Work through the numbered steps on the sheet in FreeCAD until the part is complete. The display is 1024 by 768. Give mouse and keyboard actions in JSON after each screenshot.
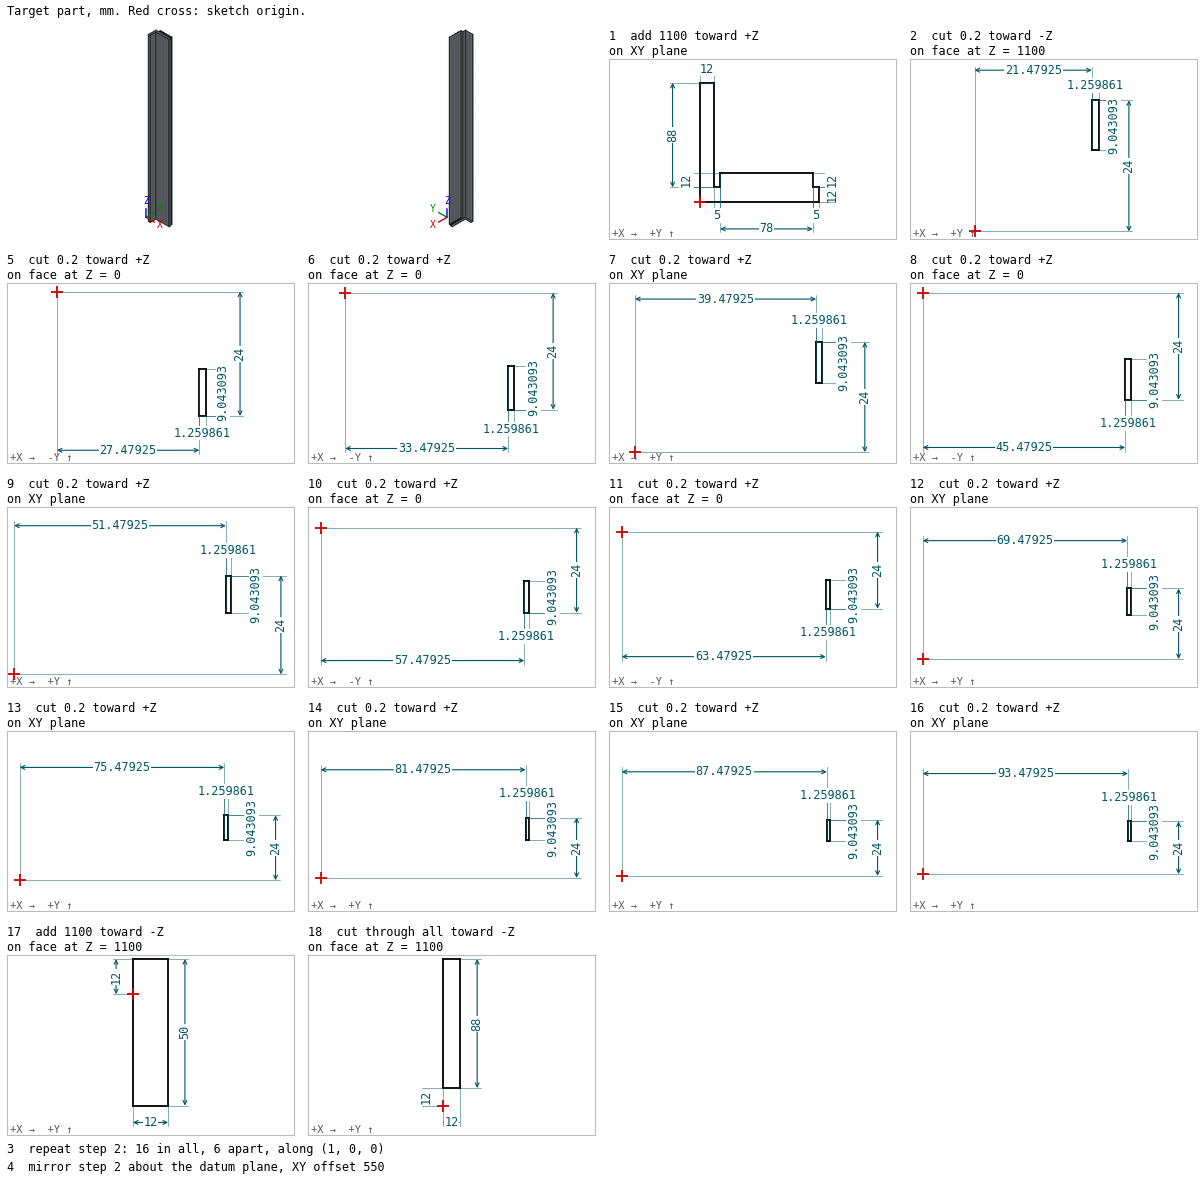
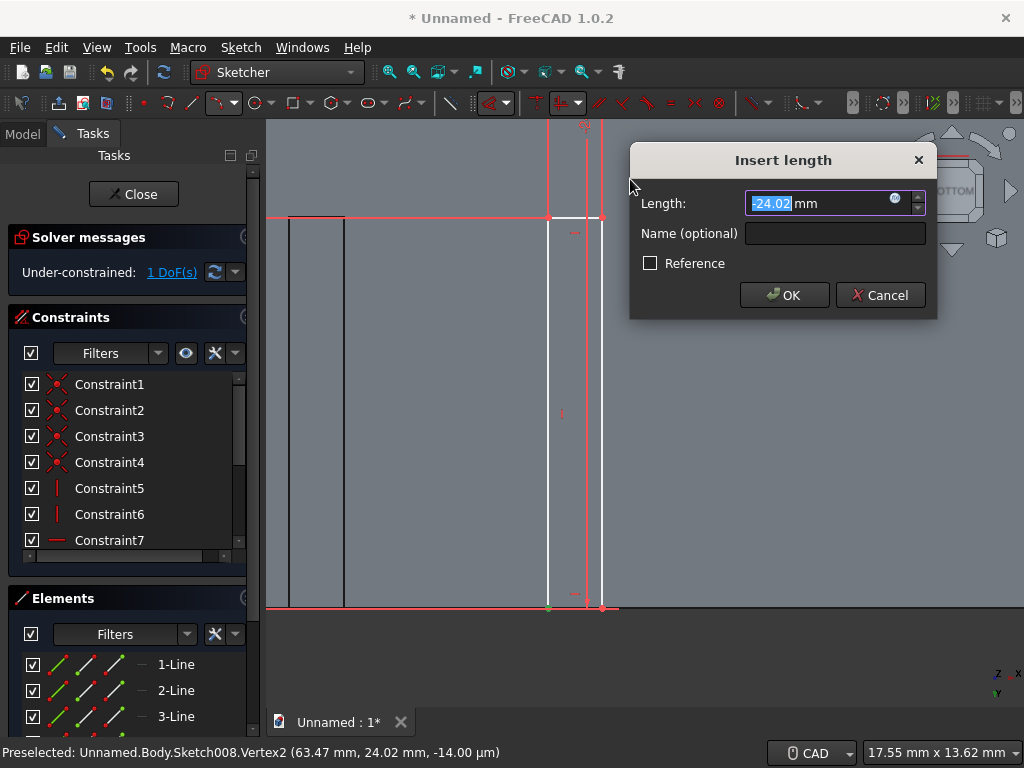
{"action": "type", "text": "-24"}
{"action": "key", "text": "Return"}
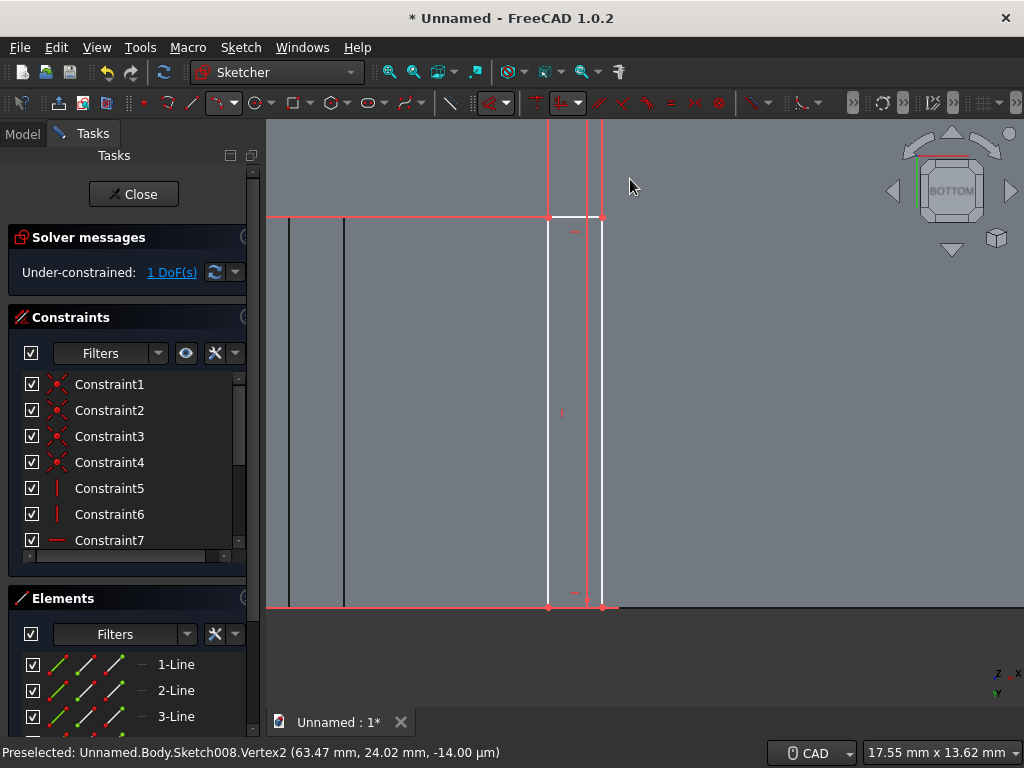
{"action": "left_click", "coordinate": [548, 217]}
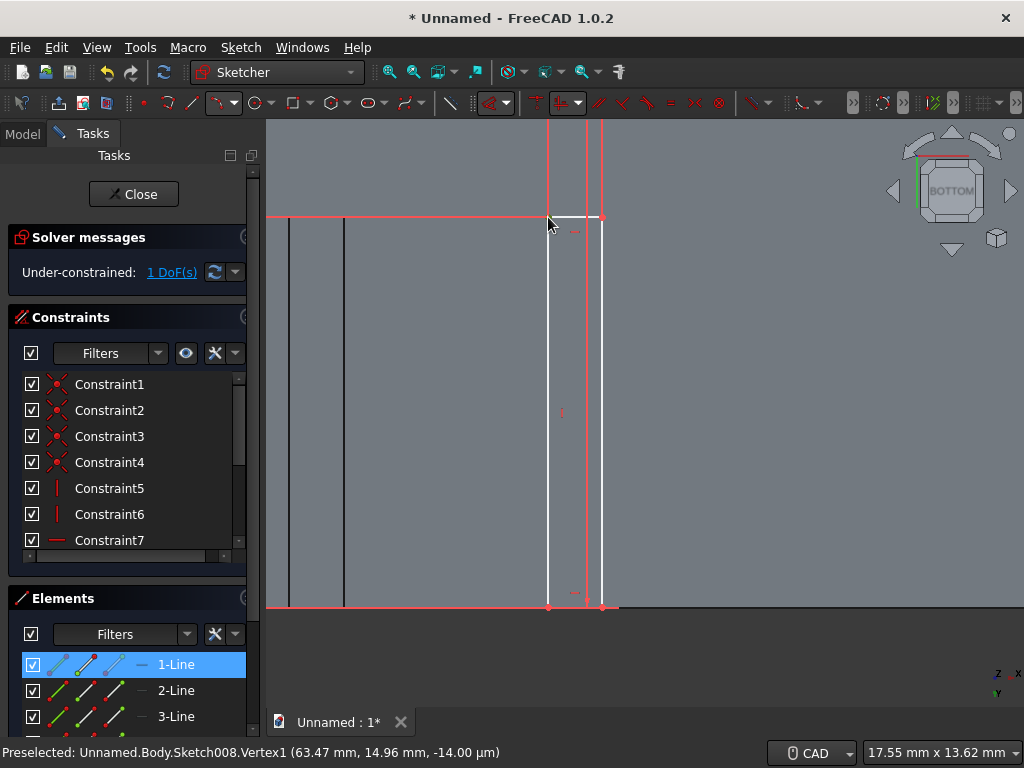
{"action": "key", "text": "l"}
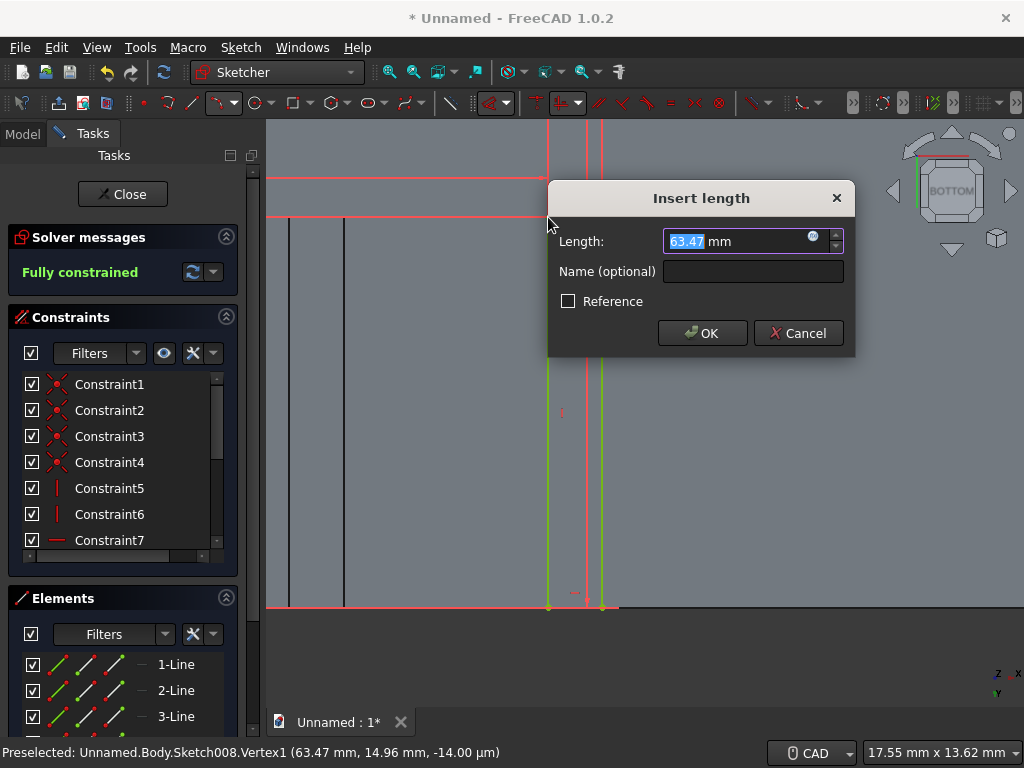
{"action": "type", "text": "63.47925"}
{"action": "key", "text": "Return"}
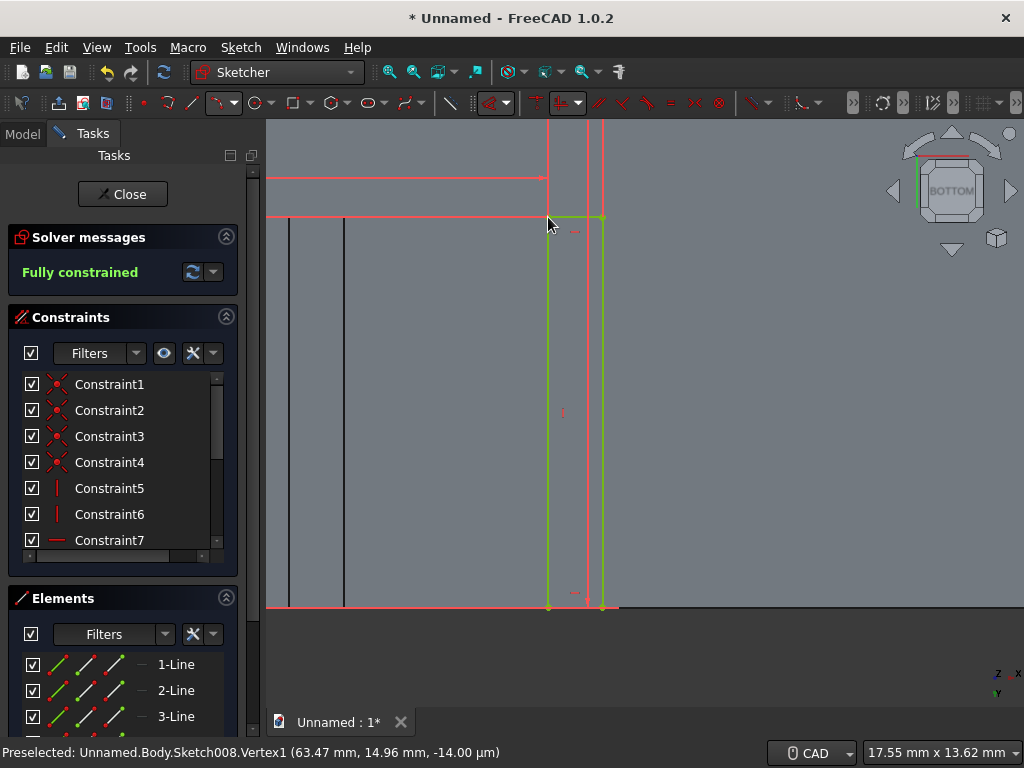
{"action": "left_click", "coordinate": [123, 194]}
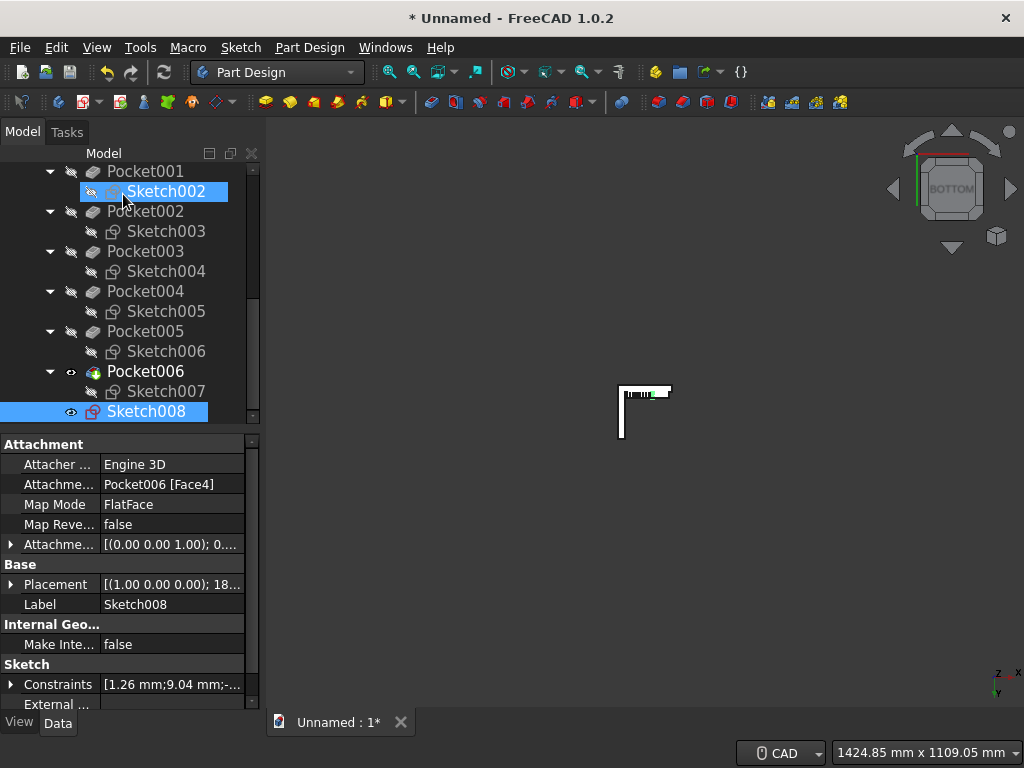
{"action": "left_click", "coordinate": [432, 102]}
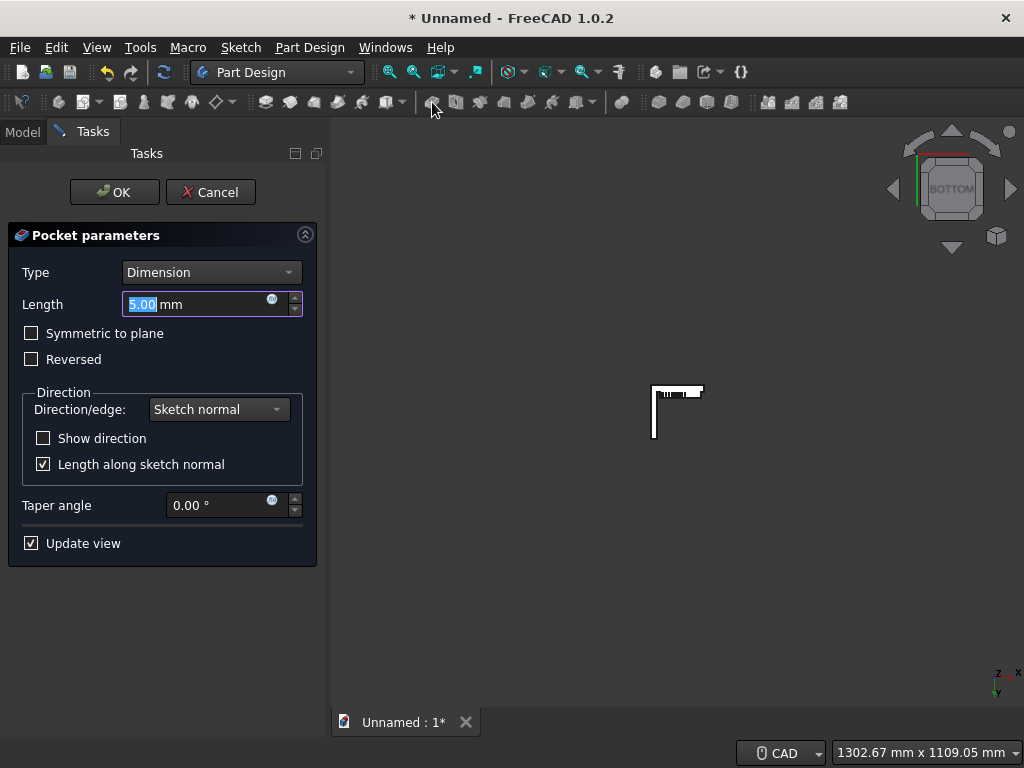
{"action": "type", "text": "0.2"}
{"action": "key", "text": "Tab"}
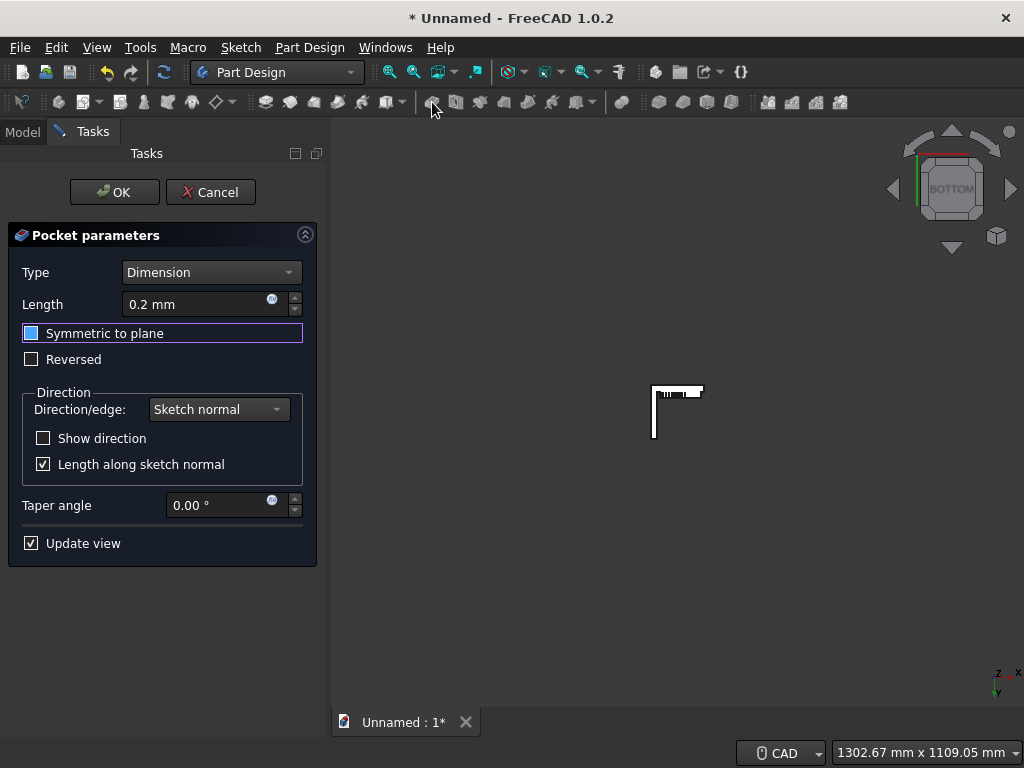
{"action": "left_click", "coordinate": [115, 192]}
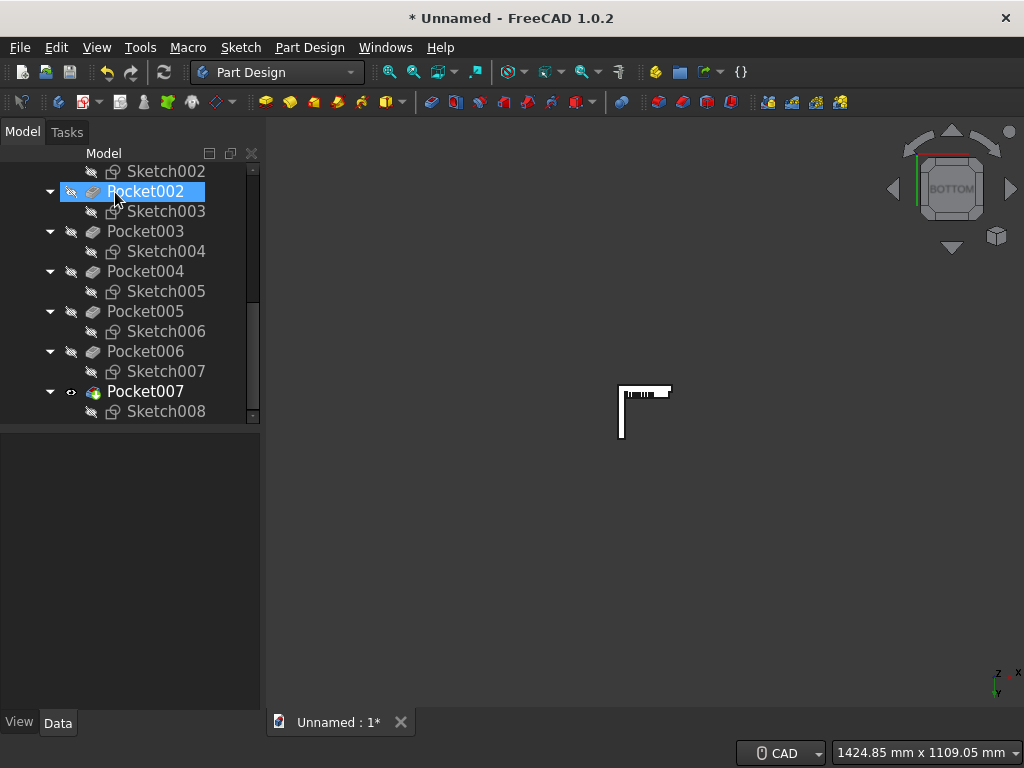
{"action": "key", "text": "v f"}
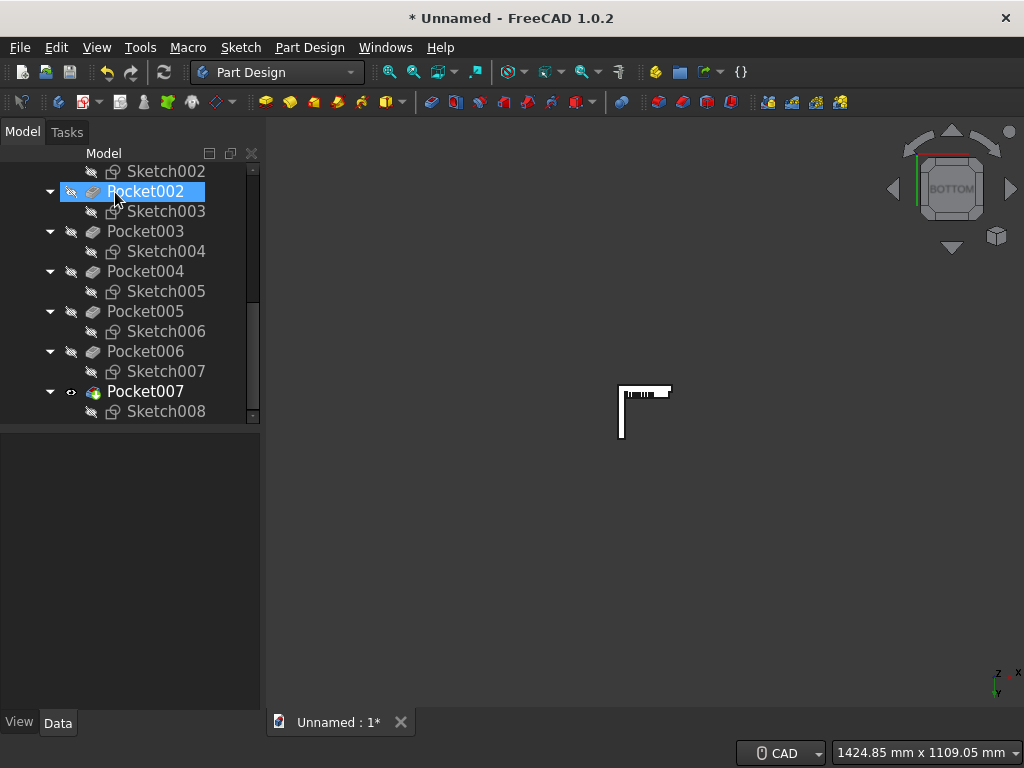
{"action": "left_click", "coordinate": [84, 102]}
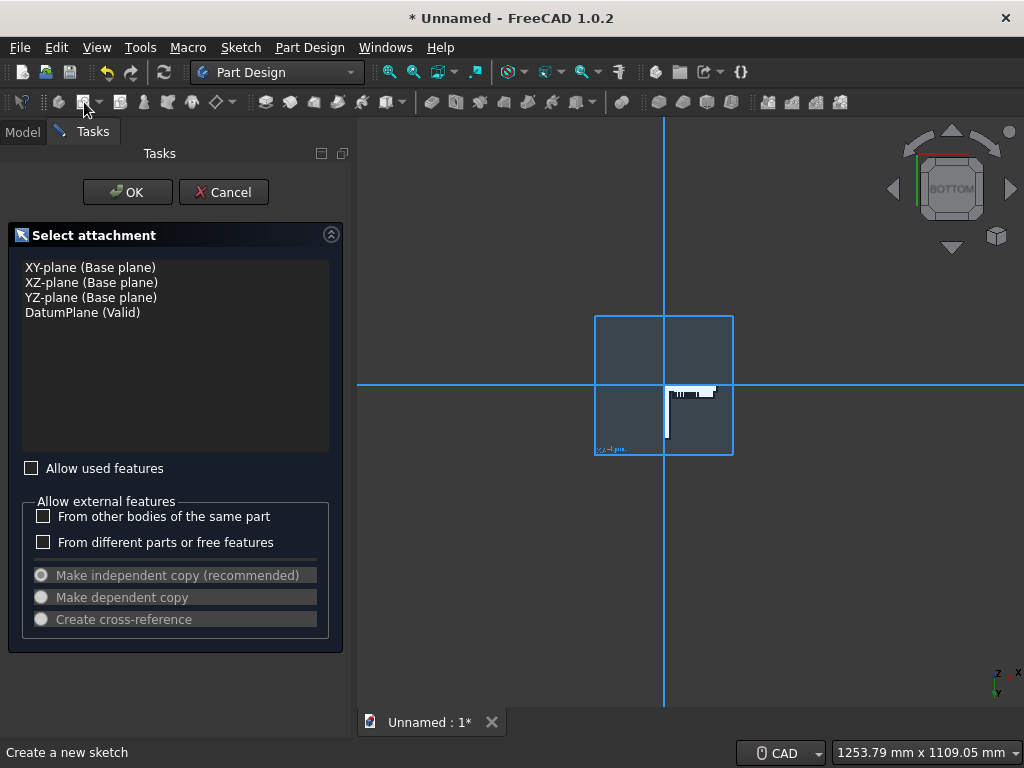
{"action": "left_click", "coordinate": [82, 268]}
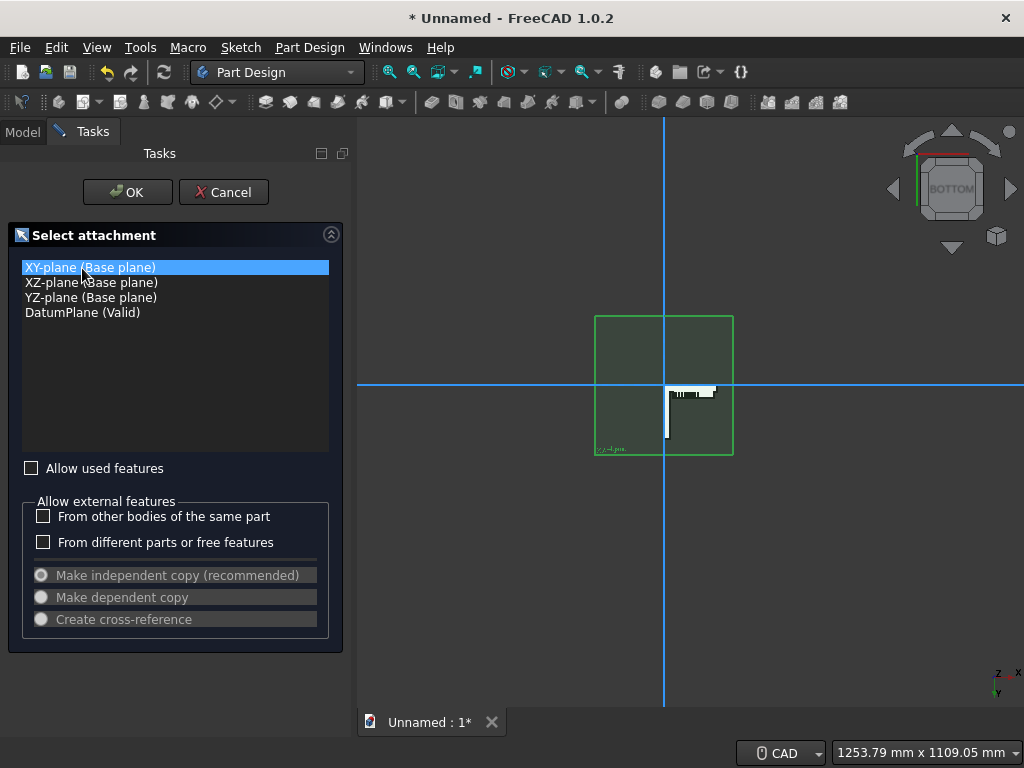
{"action": "left_click", "coordinate": [128, 192]}